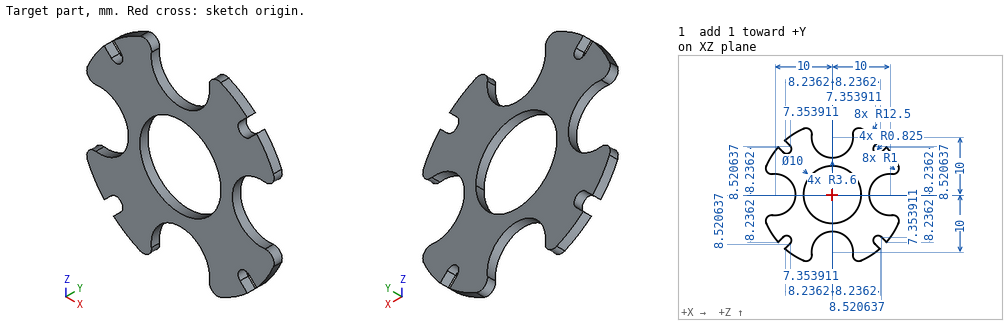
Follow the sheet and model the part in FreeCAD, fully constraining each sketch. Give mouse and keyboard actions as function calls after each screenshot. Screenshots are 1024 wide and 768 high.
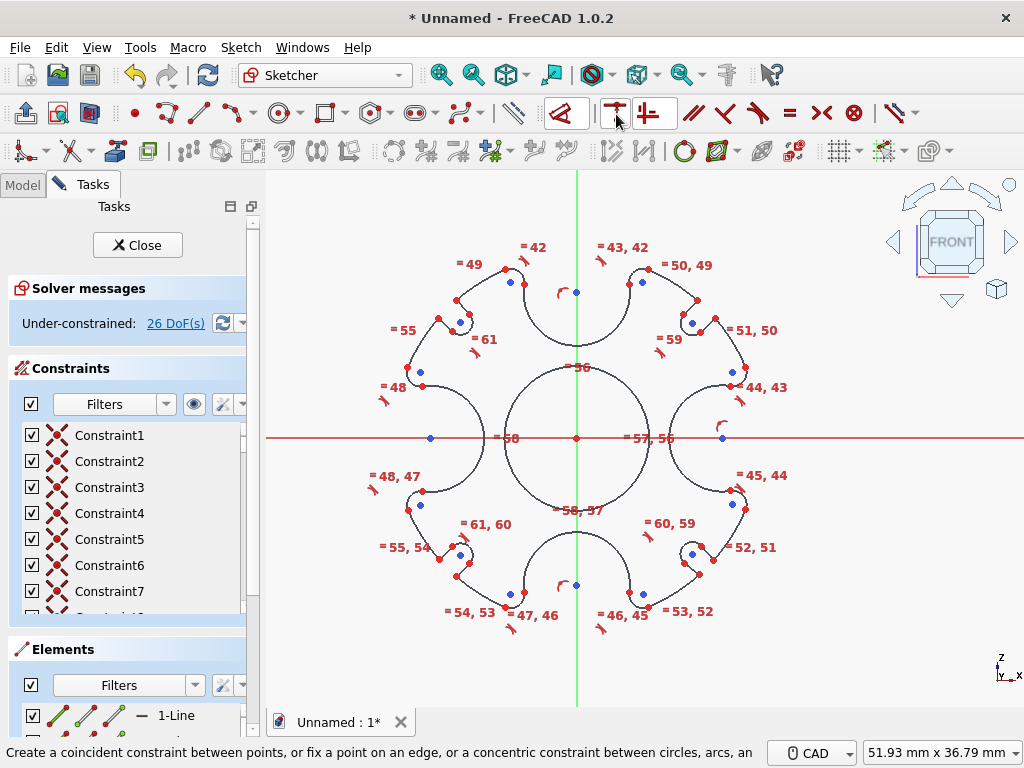
click(431, 439)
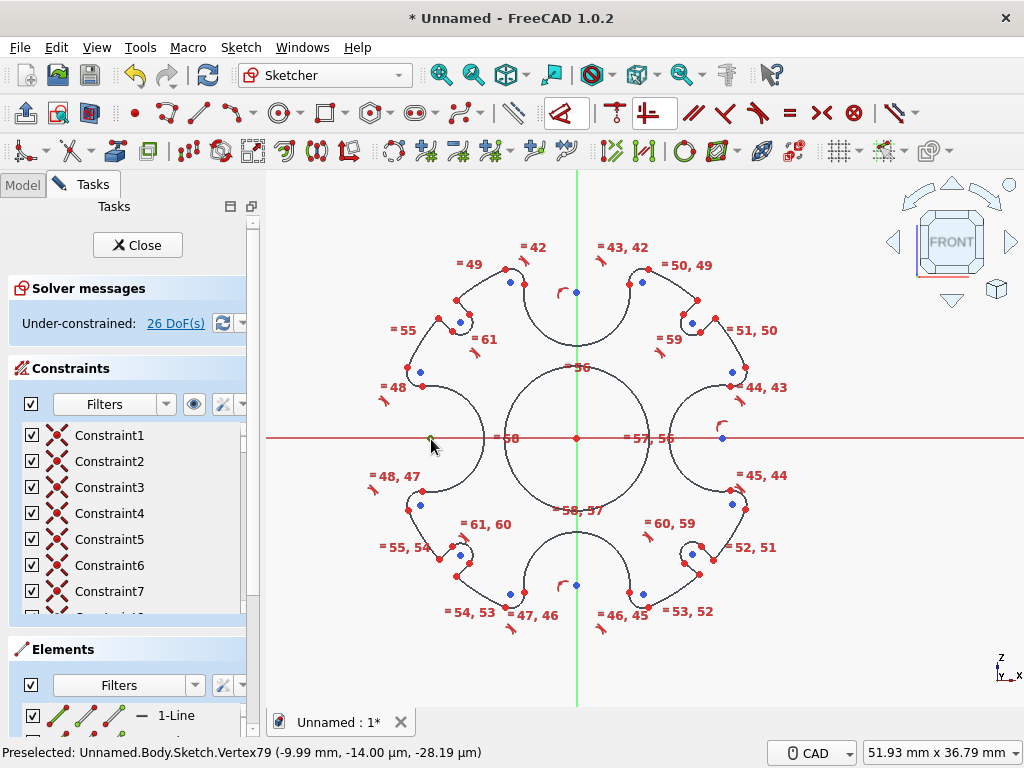
click(334, 438)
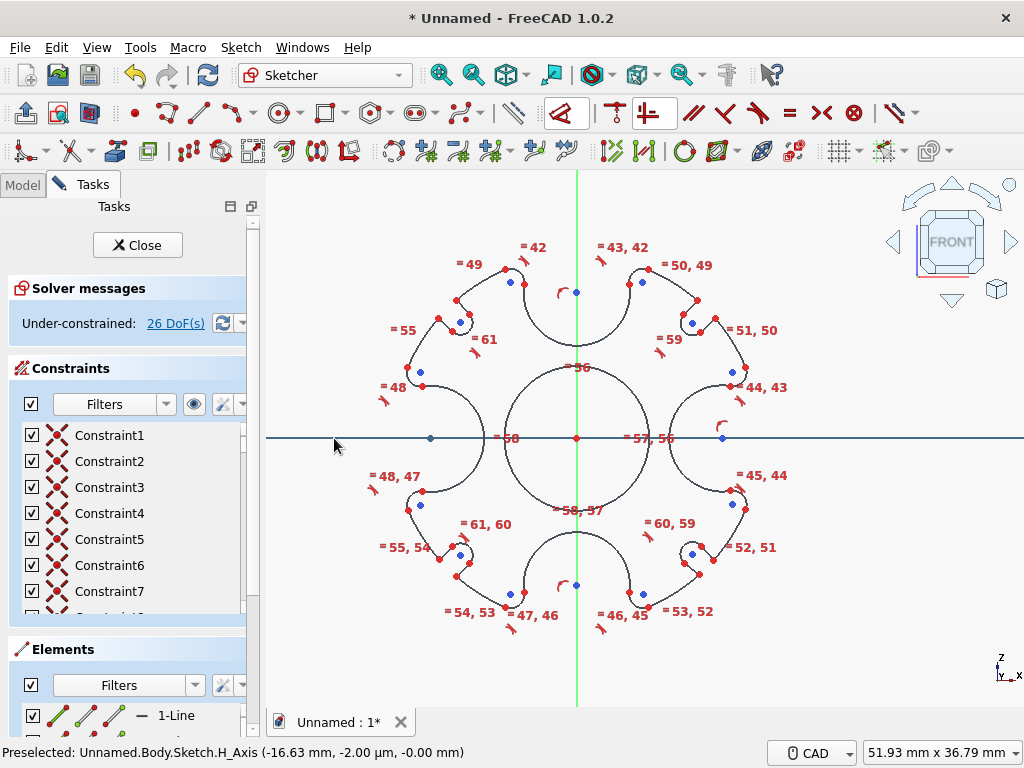
click(616, 114)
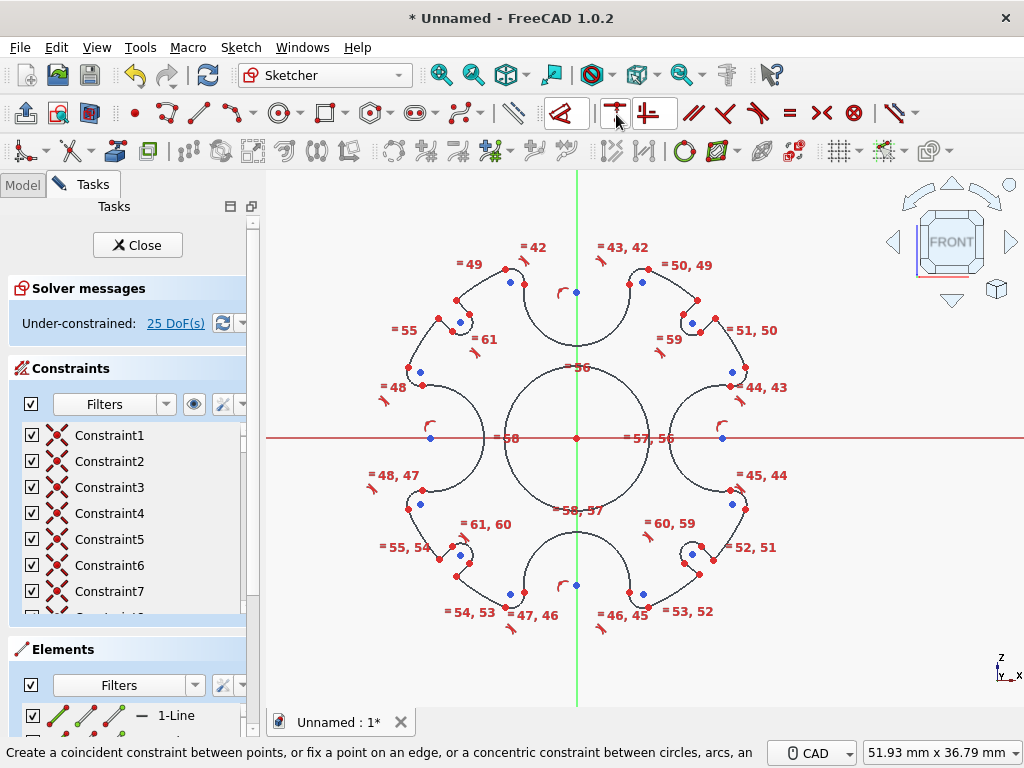
click(490, 277)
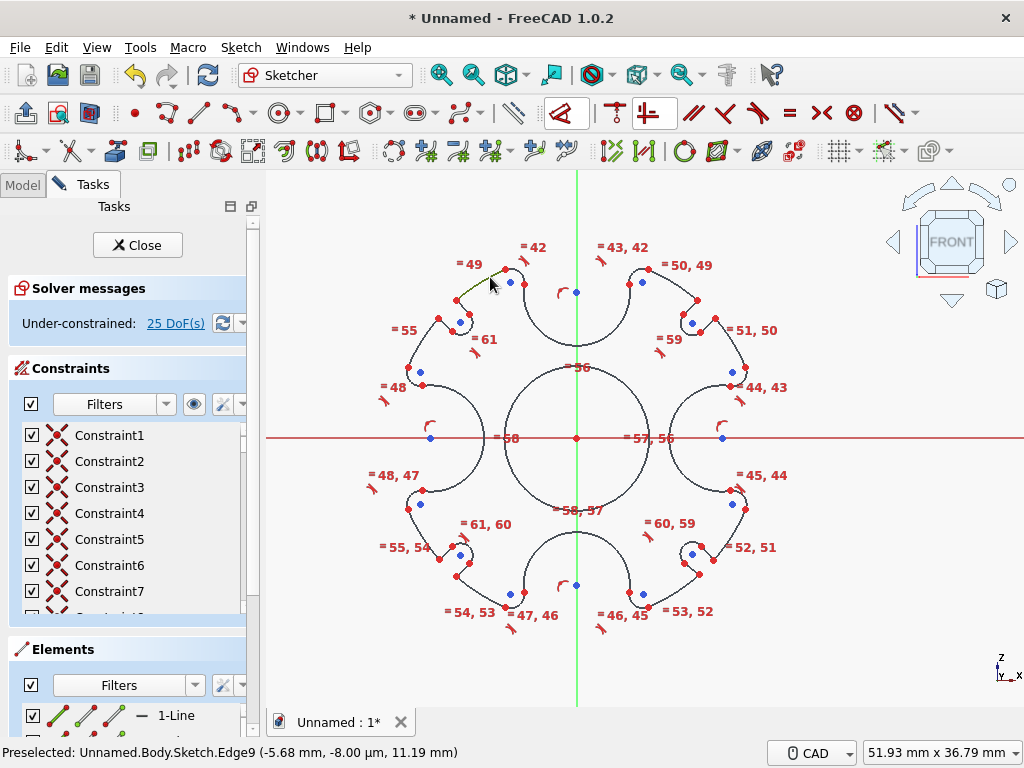
key(k)
key(r)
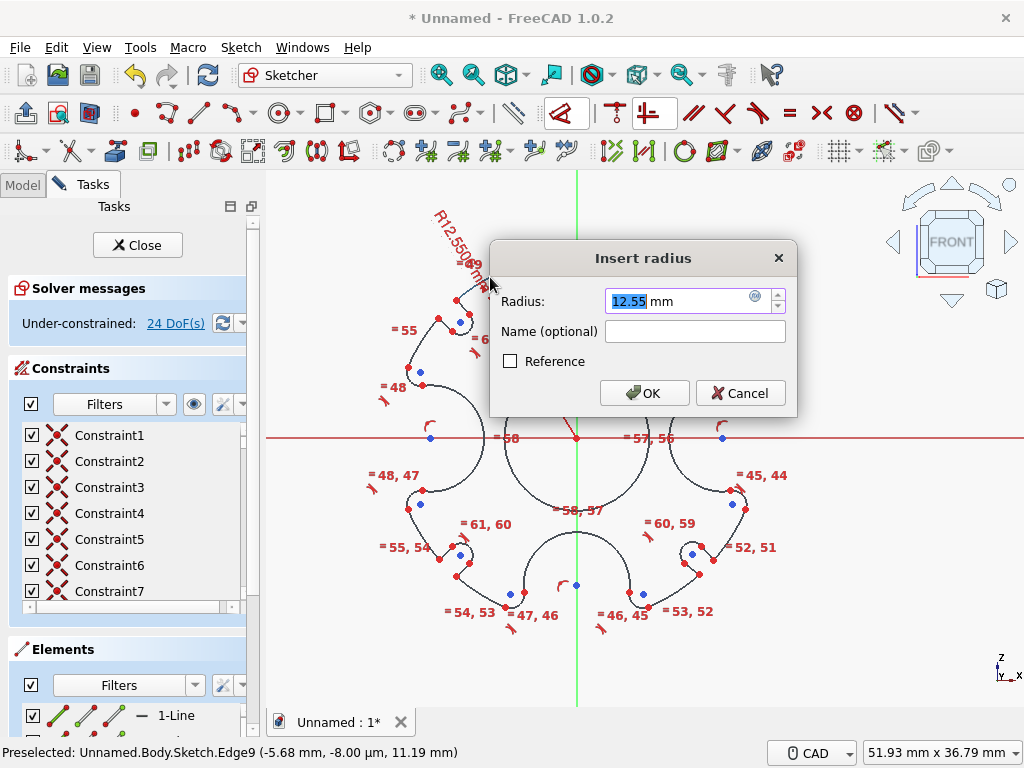
text(12.5)
key(Return)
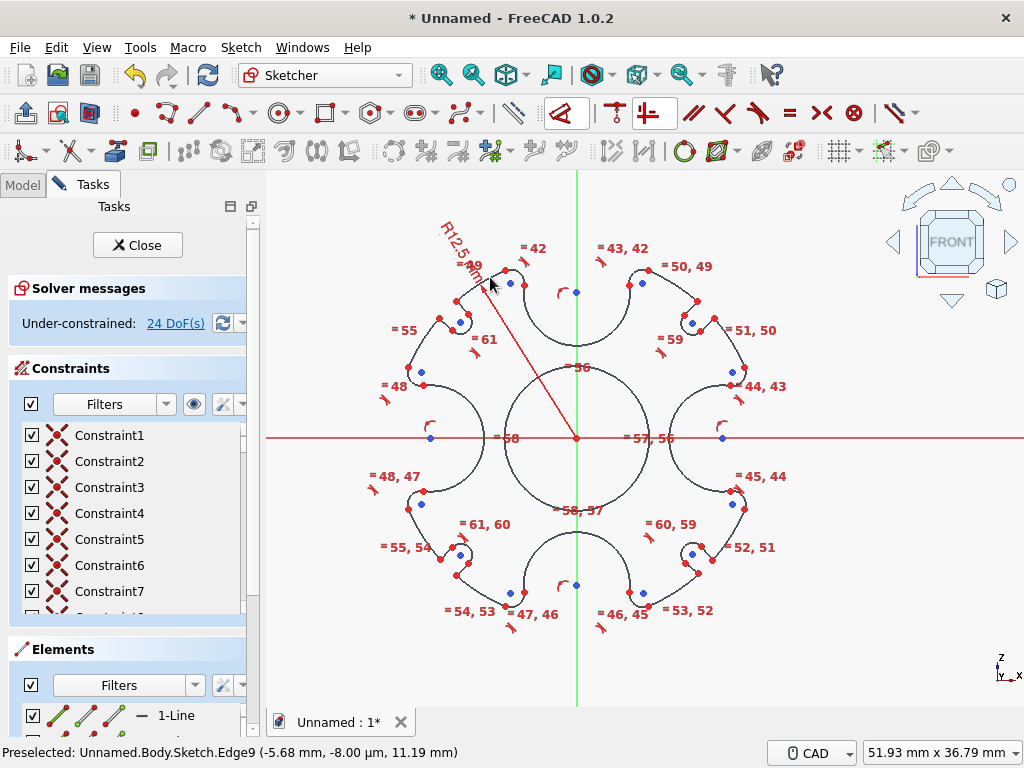
scroll(519, 272, up, 6)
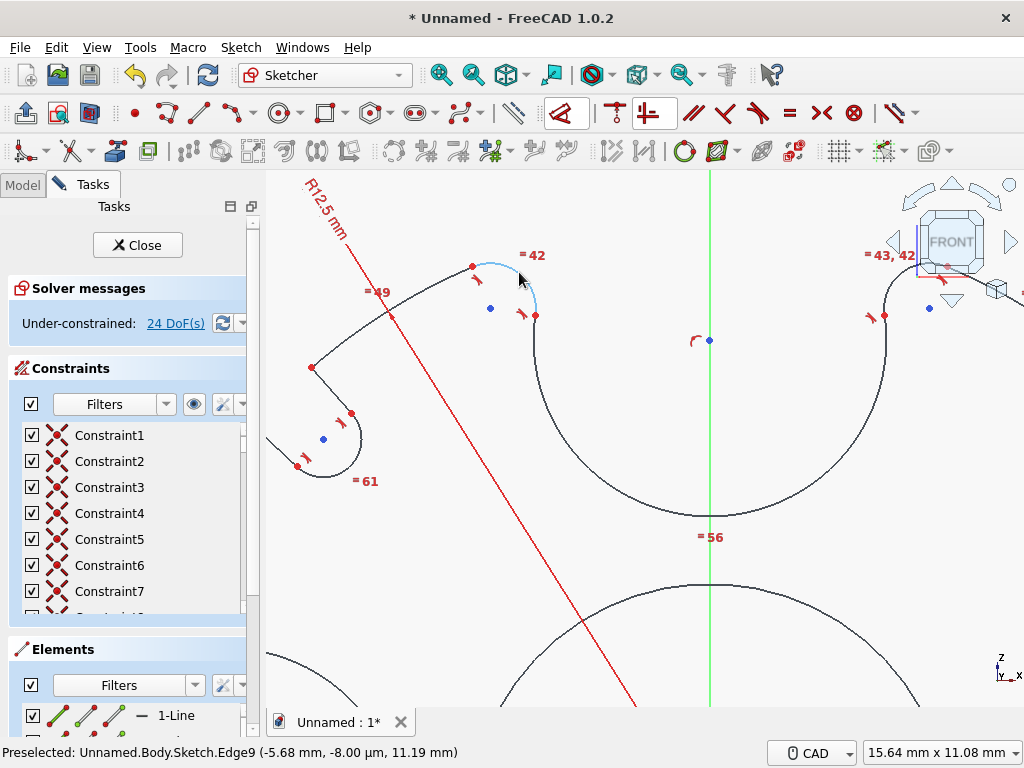
click(518, 273)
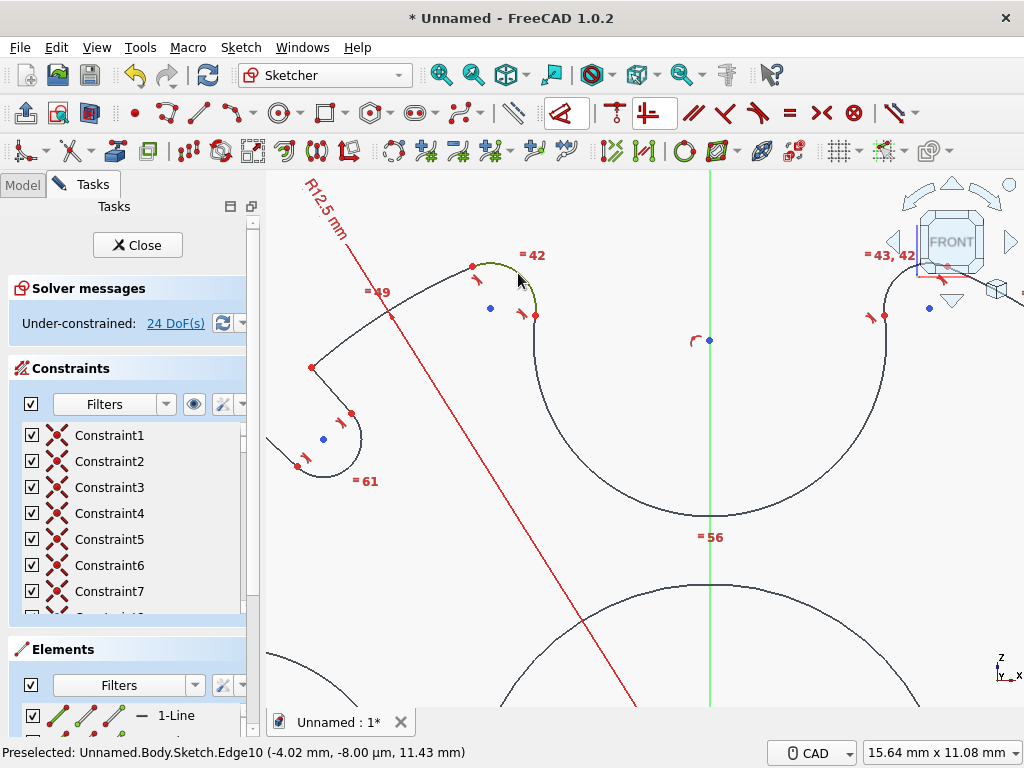
click(584, 114)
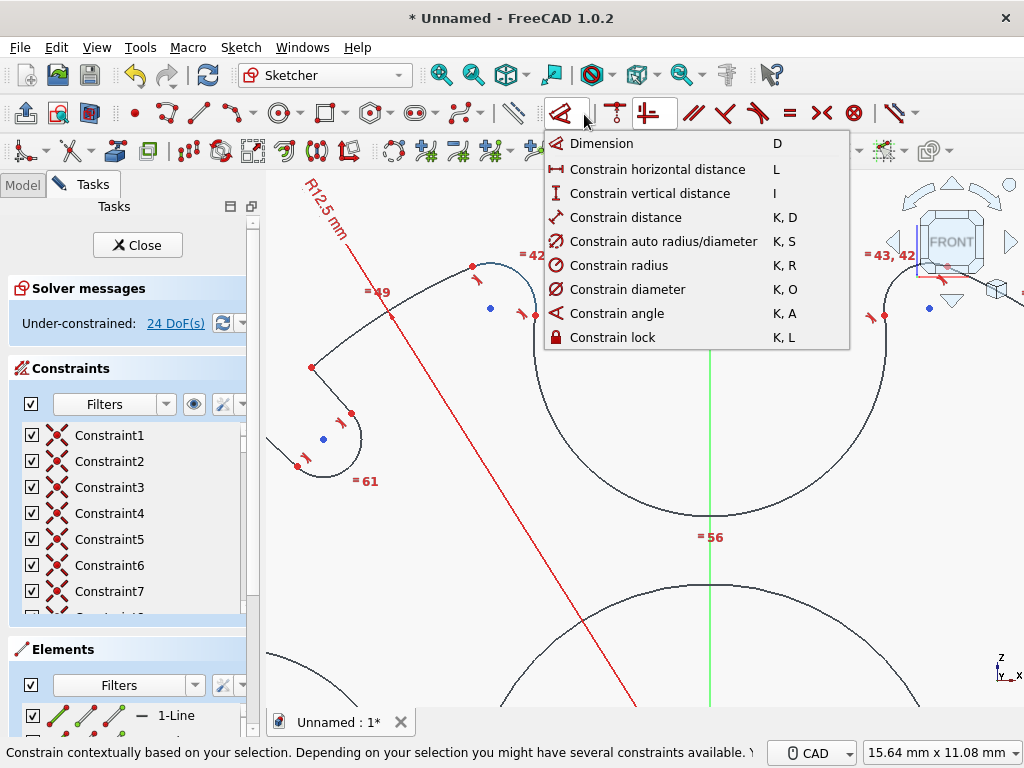
click(697, 265)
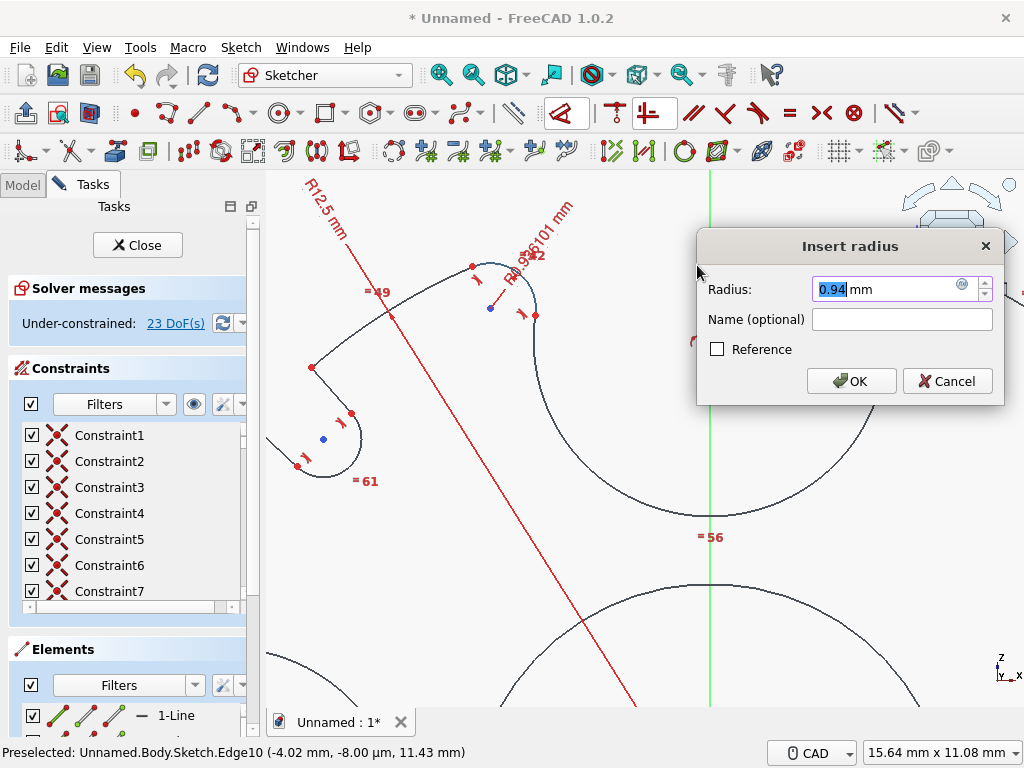
text(1)
key(Return)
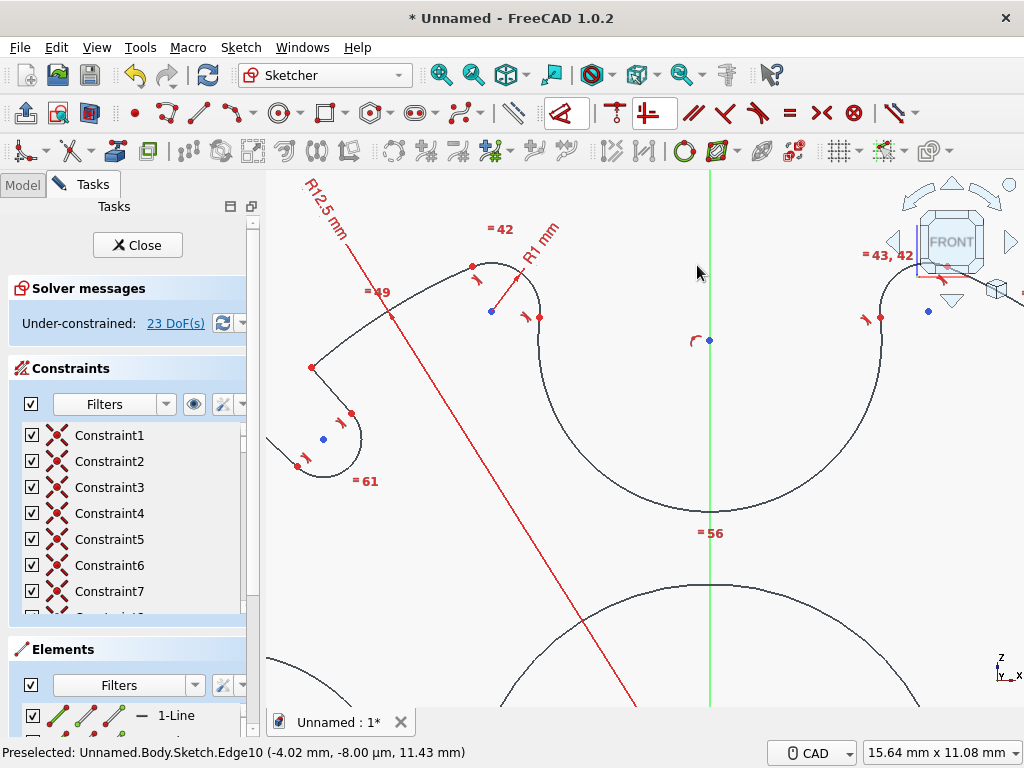
click(602, 474)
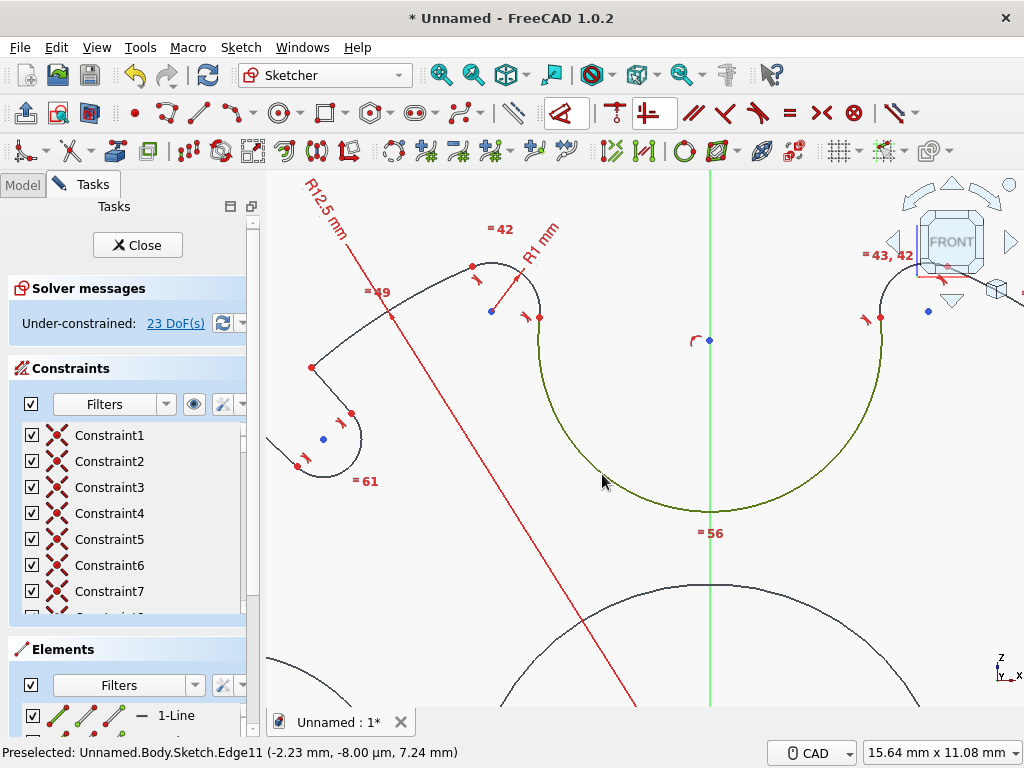
key(k)
key(r)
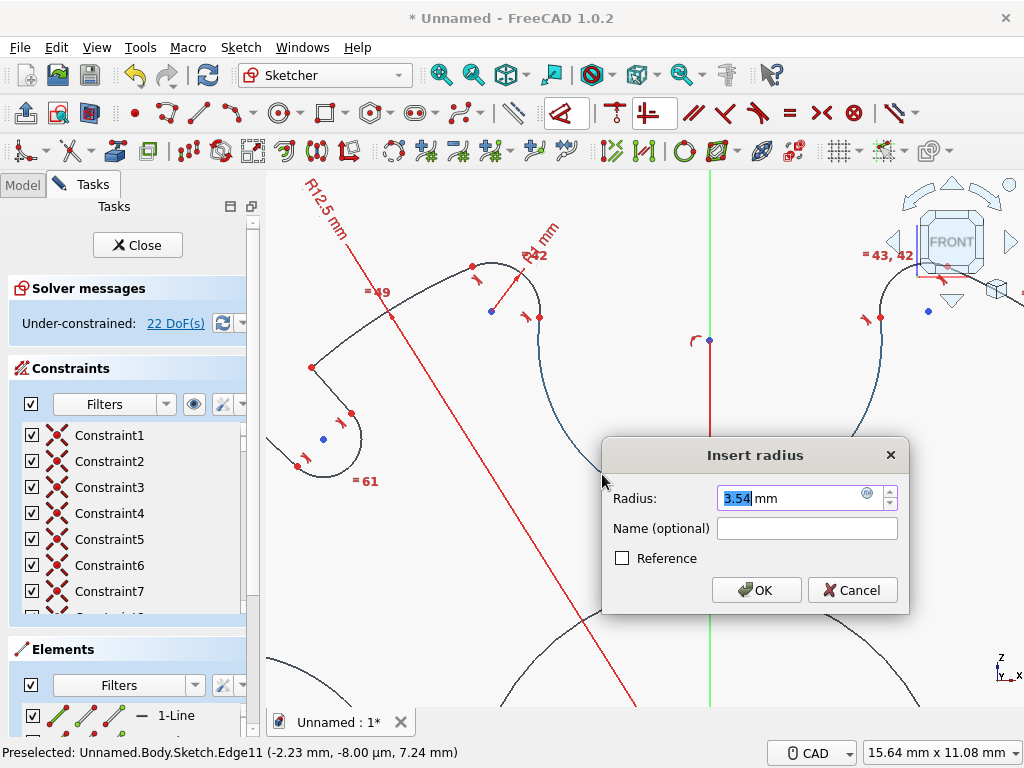
text(3.6)
key(Return)